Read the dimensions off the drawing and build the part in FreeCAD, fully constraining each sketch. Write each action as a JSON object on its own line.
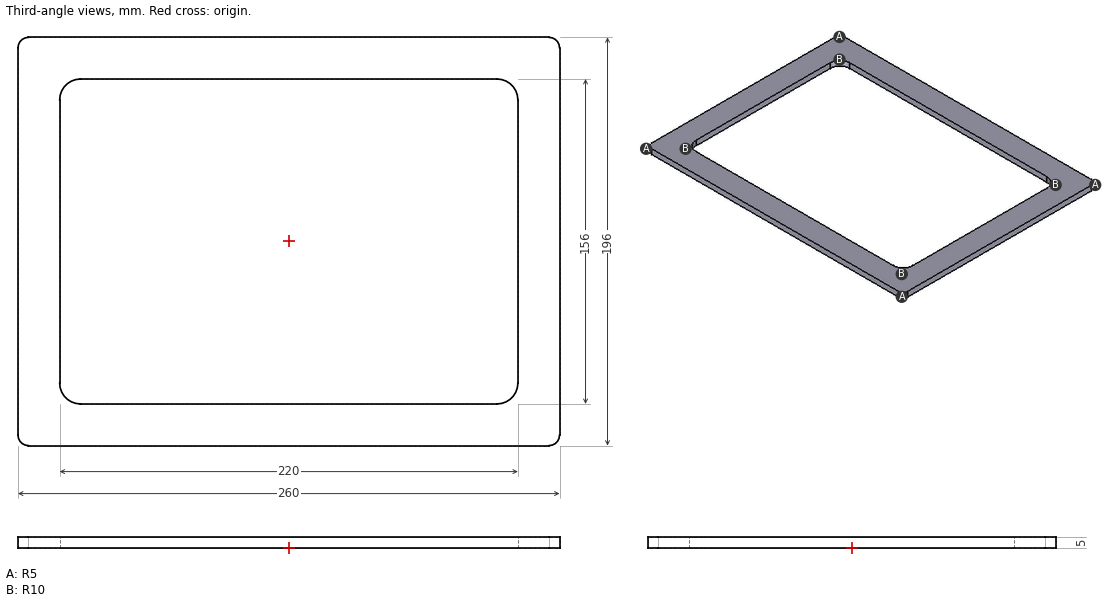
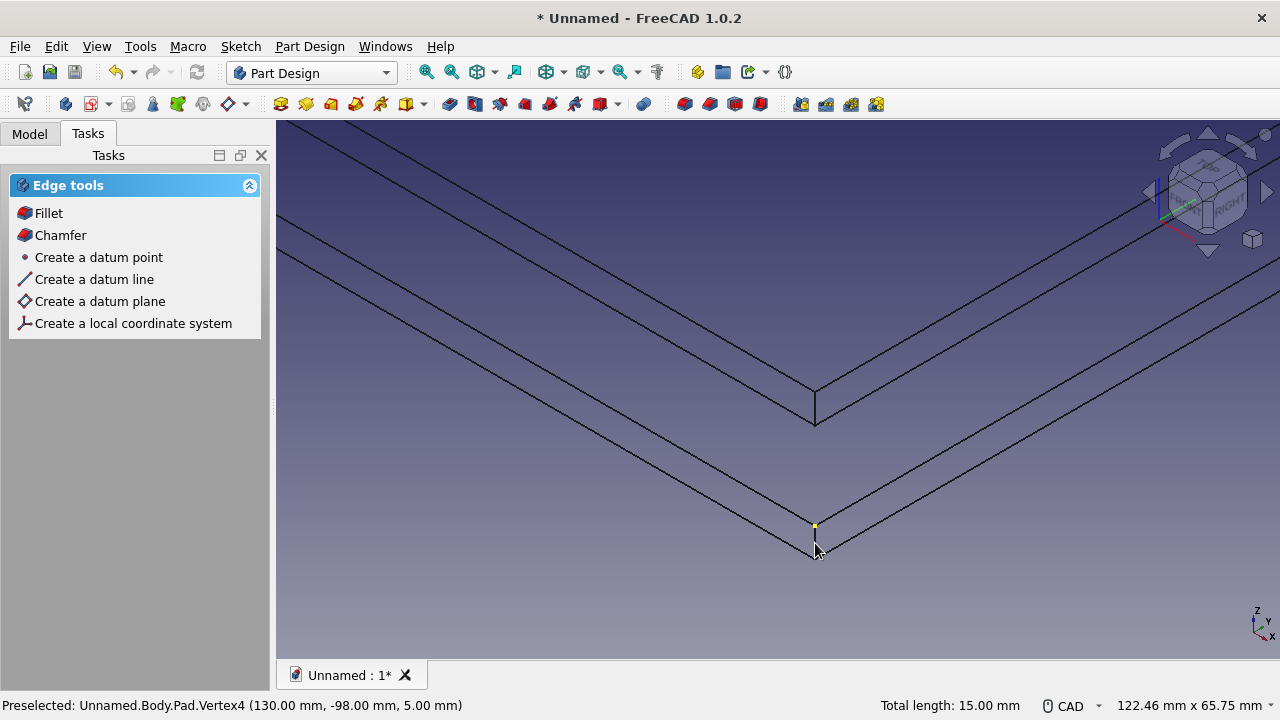
{"action": "left_click", "coordinate": [815, 542], "text": "ctrl"}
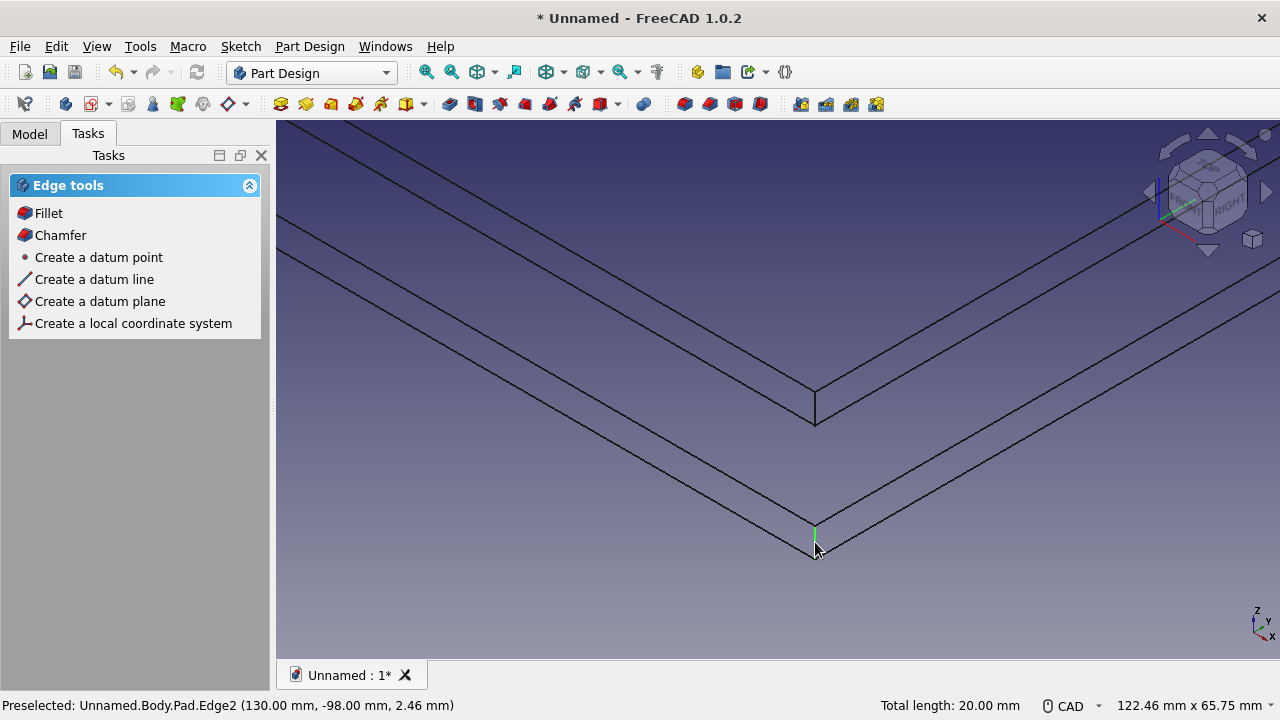
{"action": "key", "text": "v 1"}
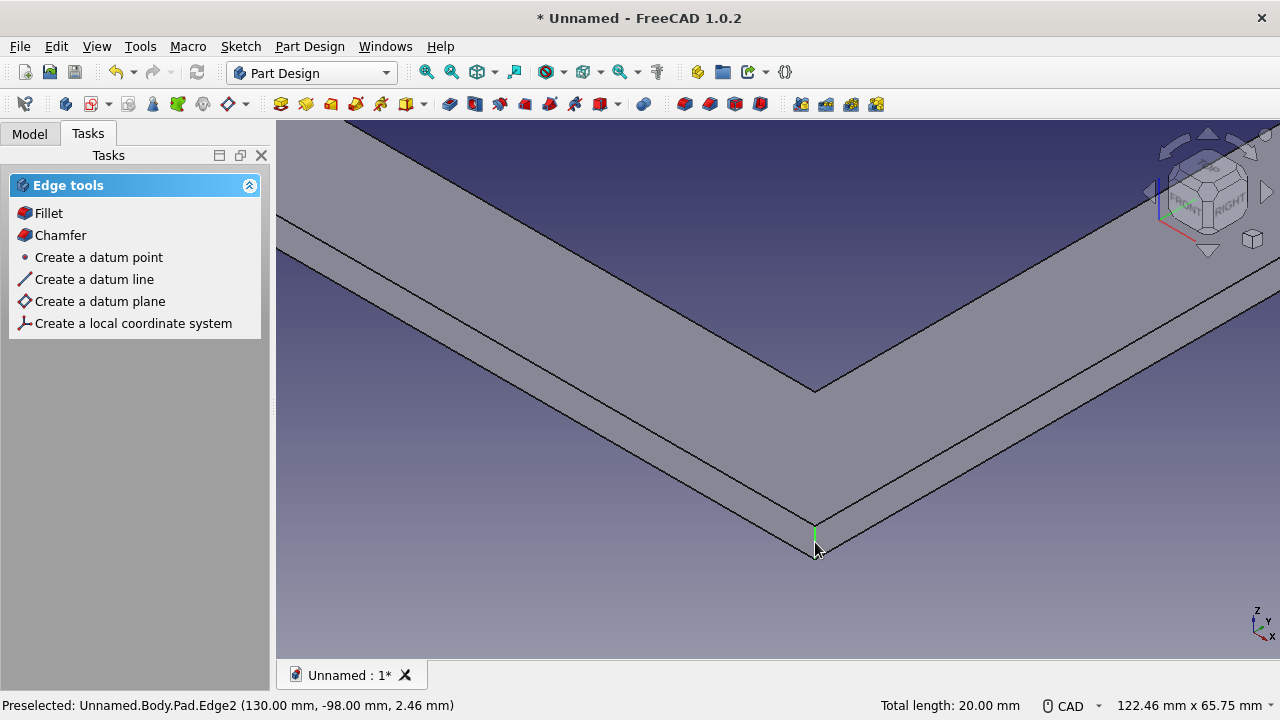
{"action": "left_click", "coordinate": [685, 104]}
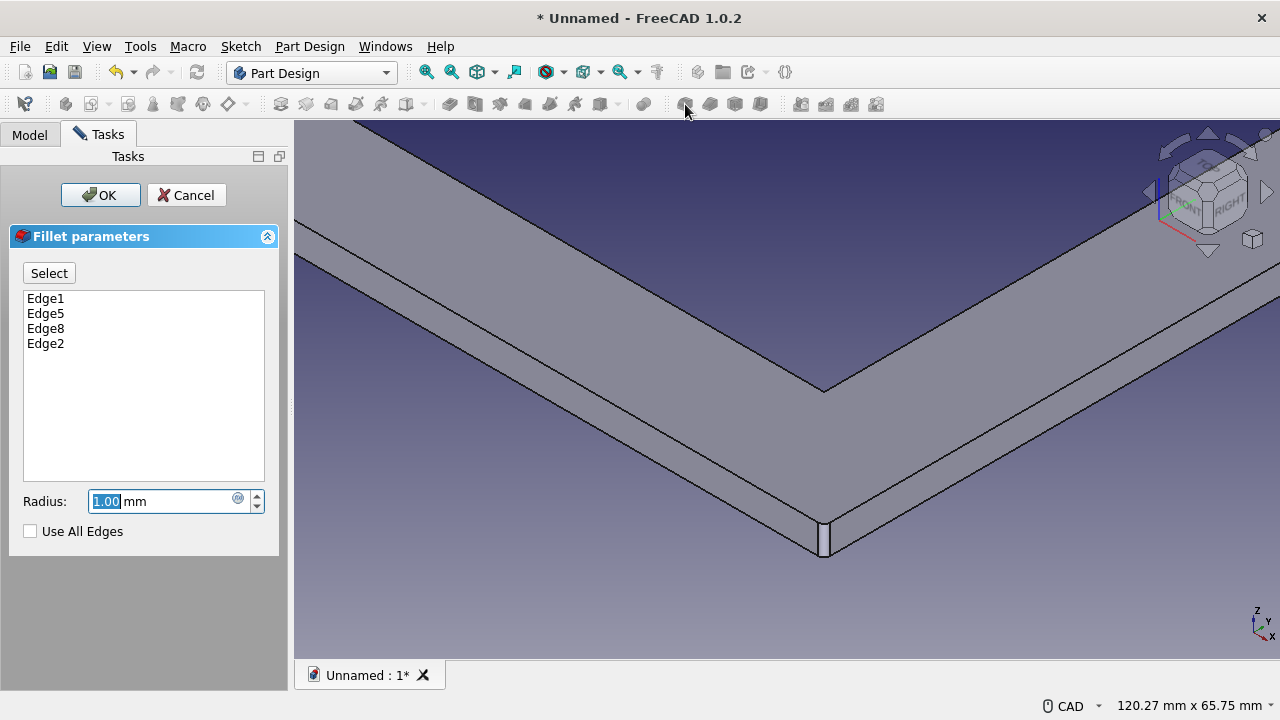
{"action": "type", "text": "5"}
{"action": "key", "text": "Tab"}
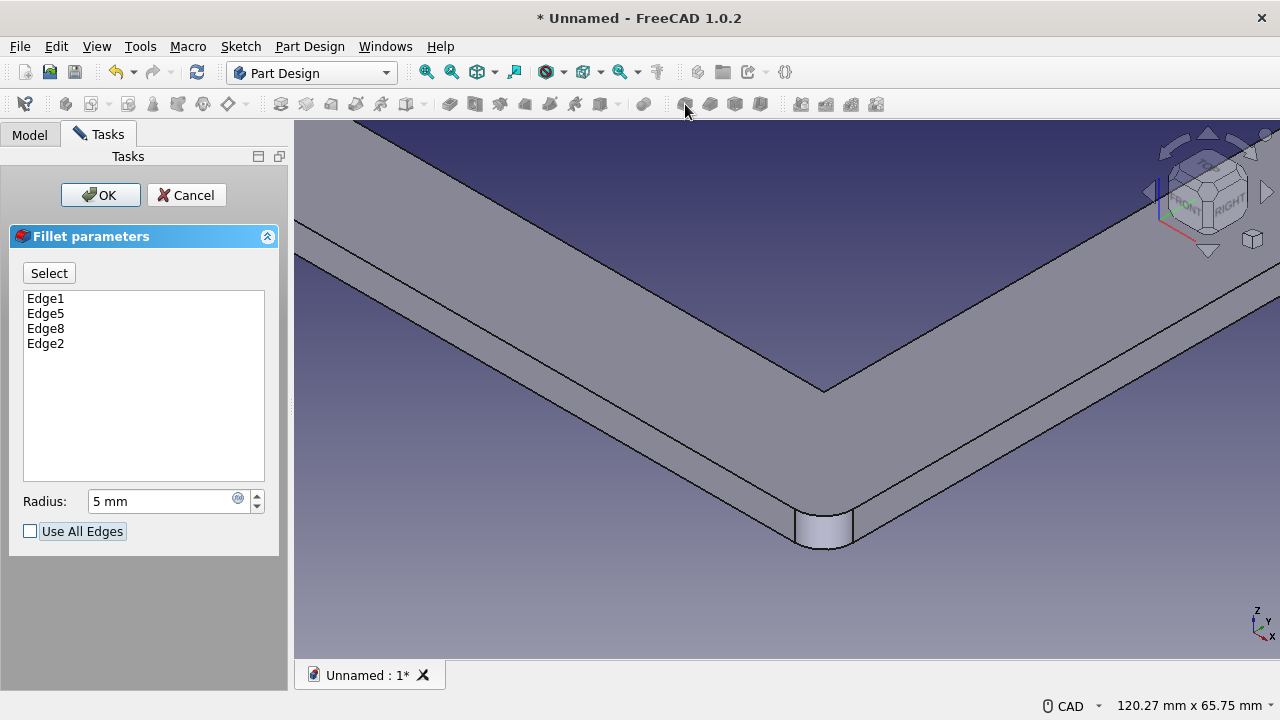
{"action": "left_click", "coordinate": [101, 195]}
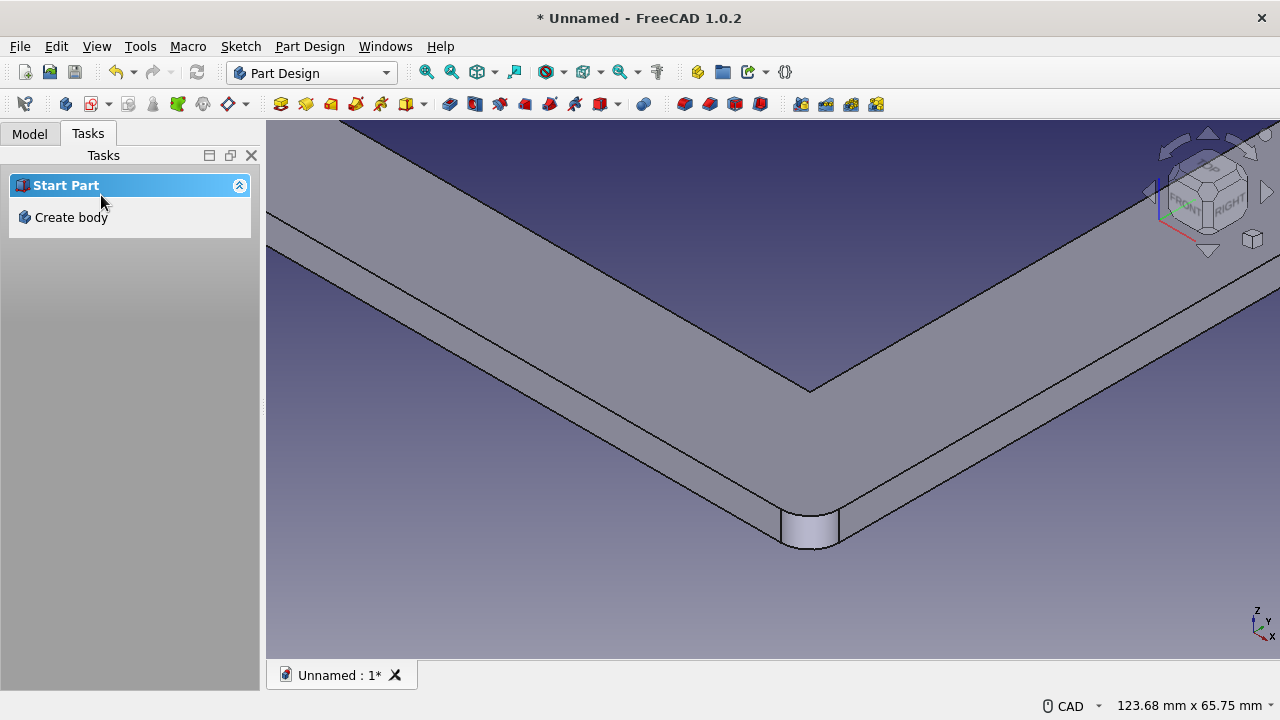
{"action": "left_click", "coordinate": [427, 72]}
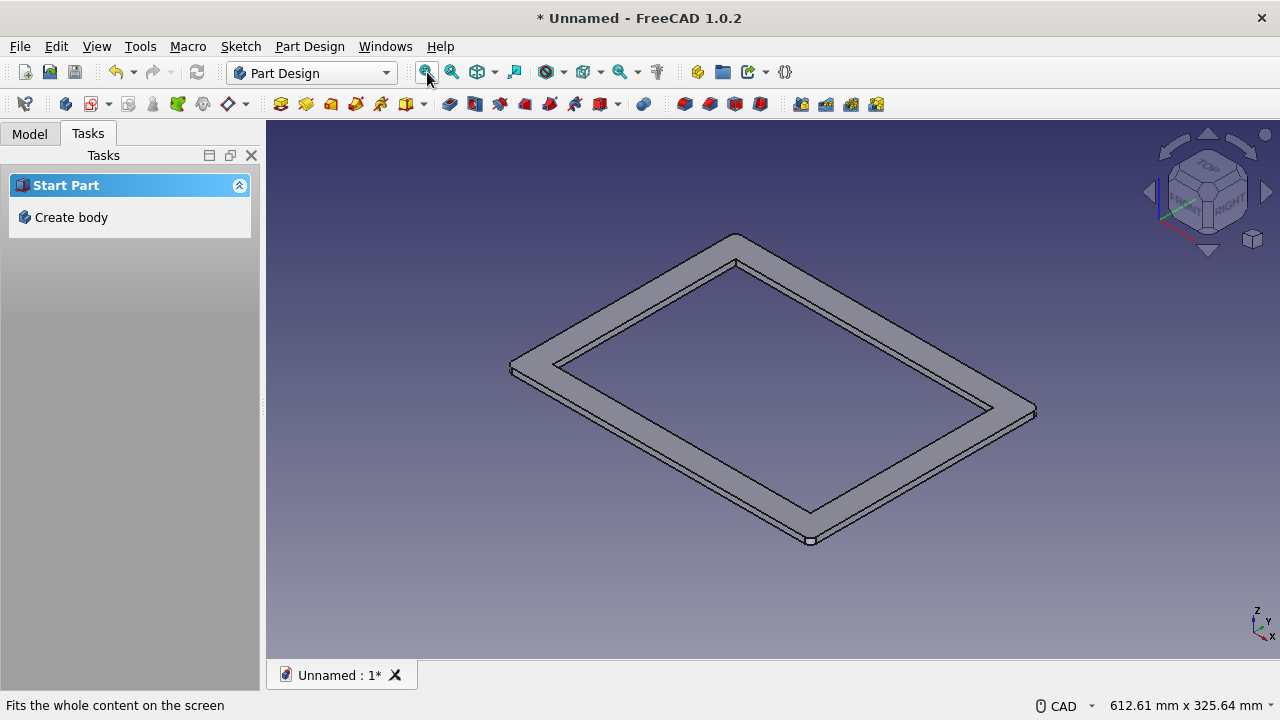
{"action": "scroll", "coordinate": [736, 261], "scroll_direction": "up", "scroll_amount": 8}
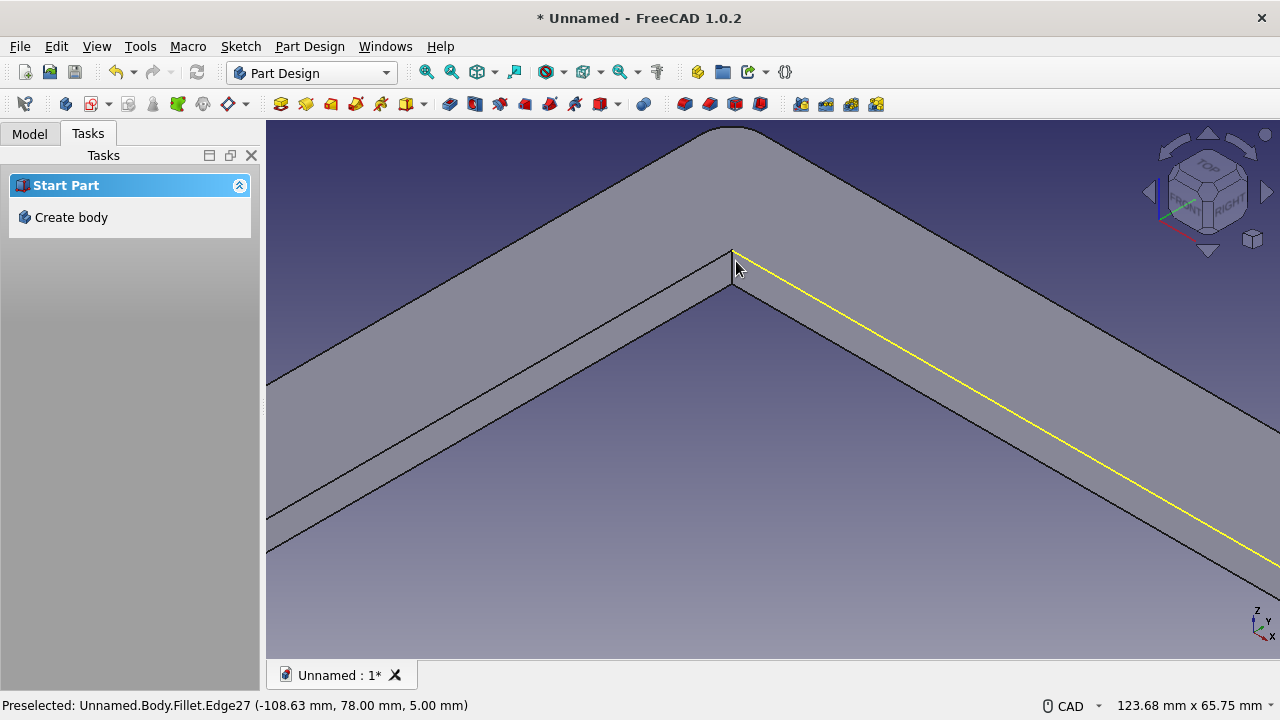
{"action": "left_click", "coordinate": [427, 72]}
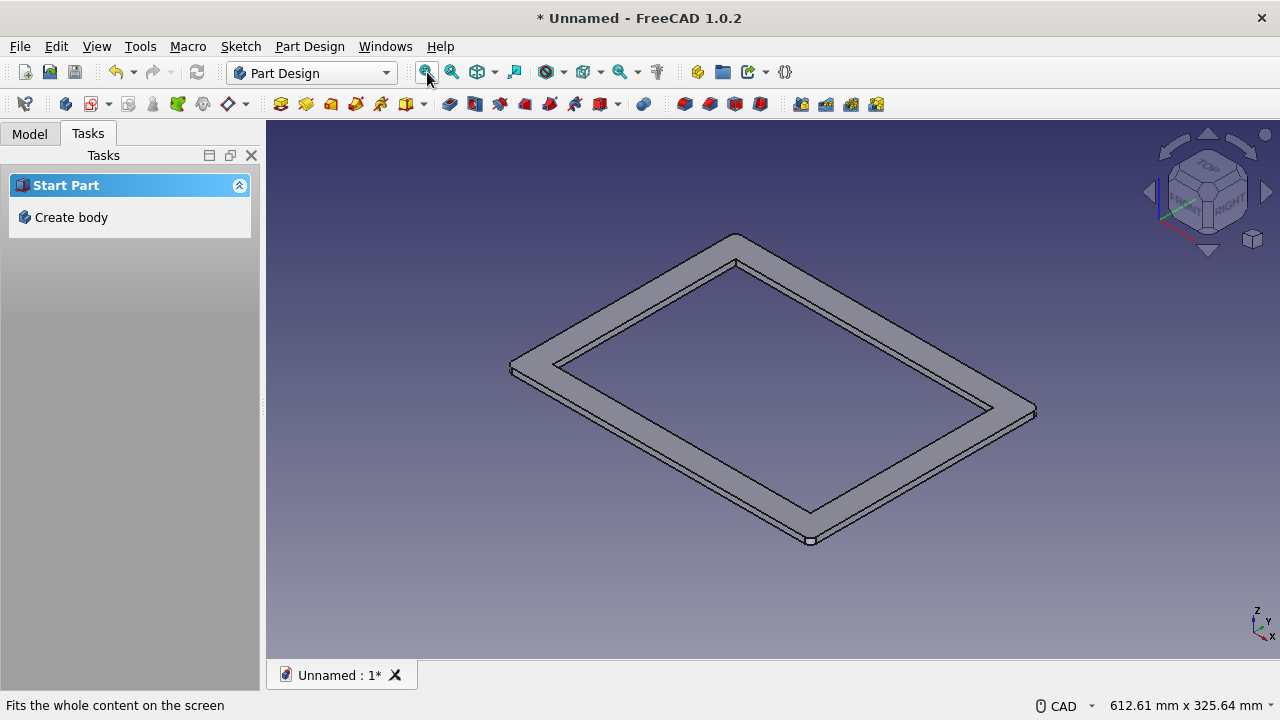
{"action": "key", "text": "2"}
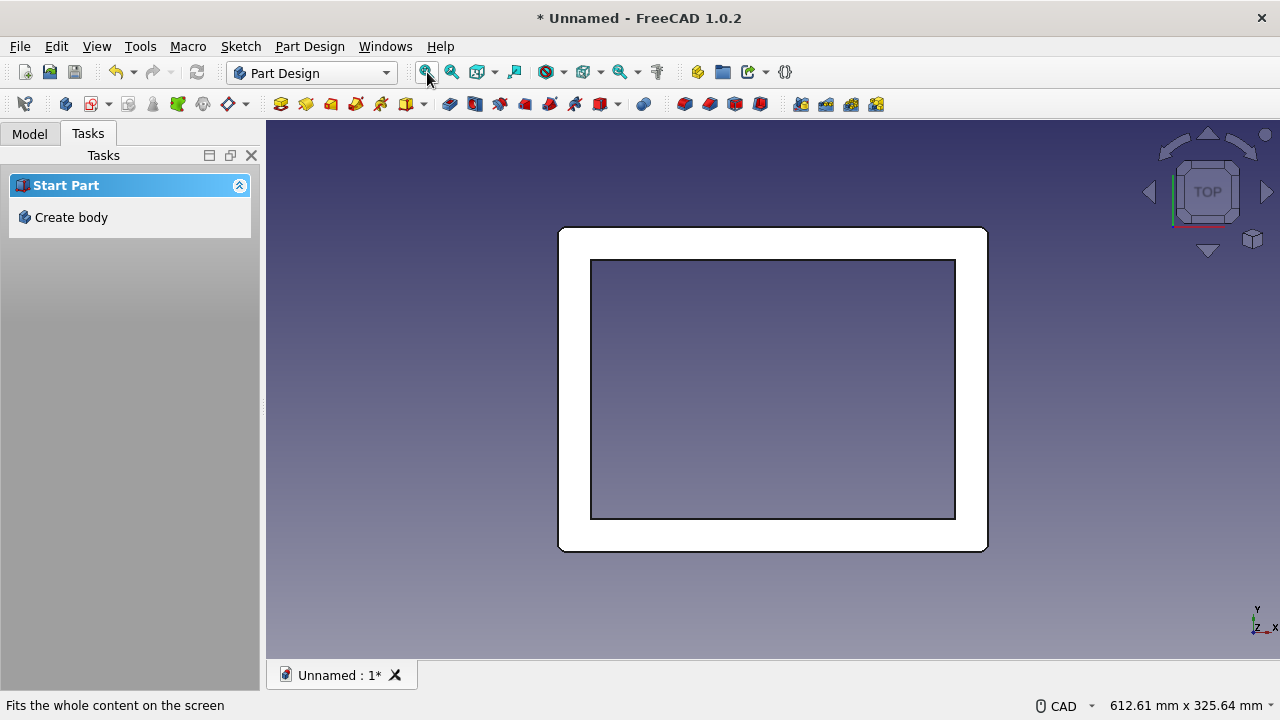
{"action": "scroll", "coordinate": [591, 259], "scroll_direction": "up", "scroll_amount": 8}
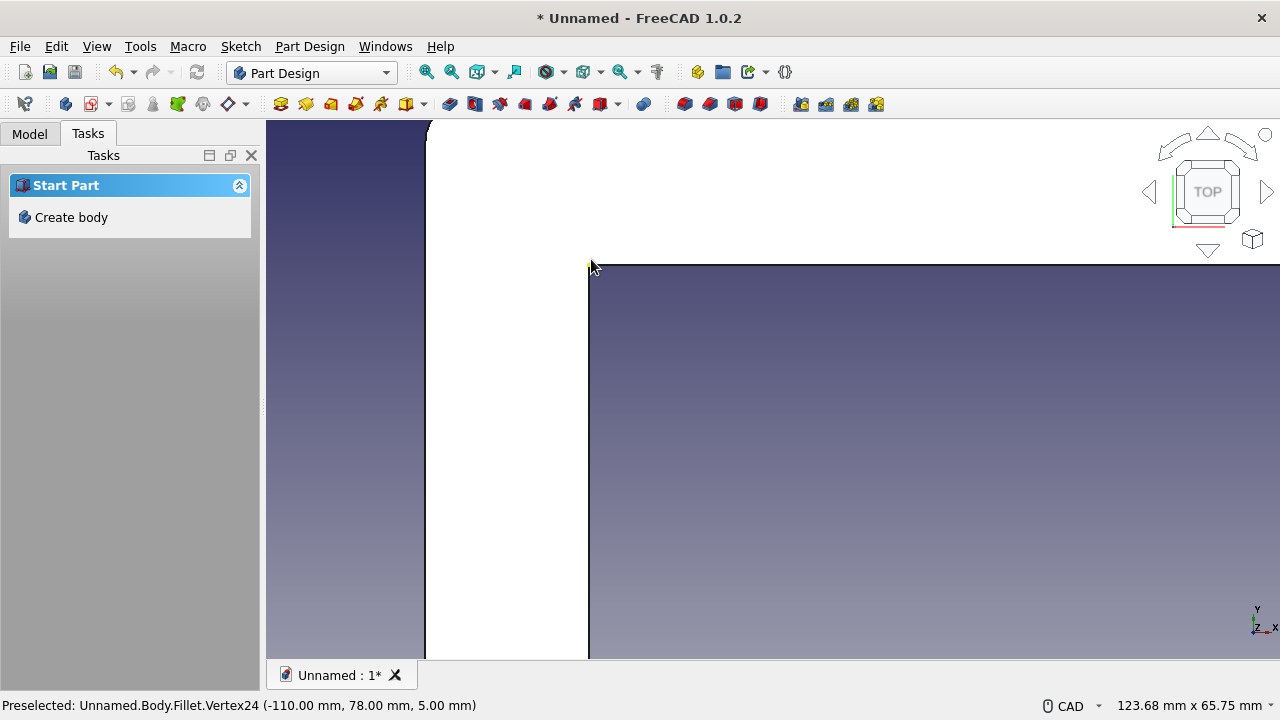
{"action": "left_click", "coordinate": [427, 72]}